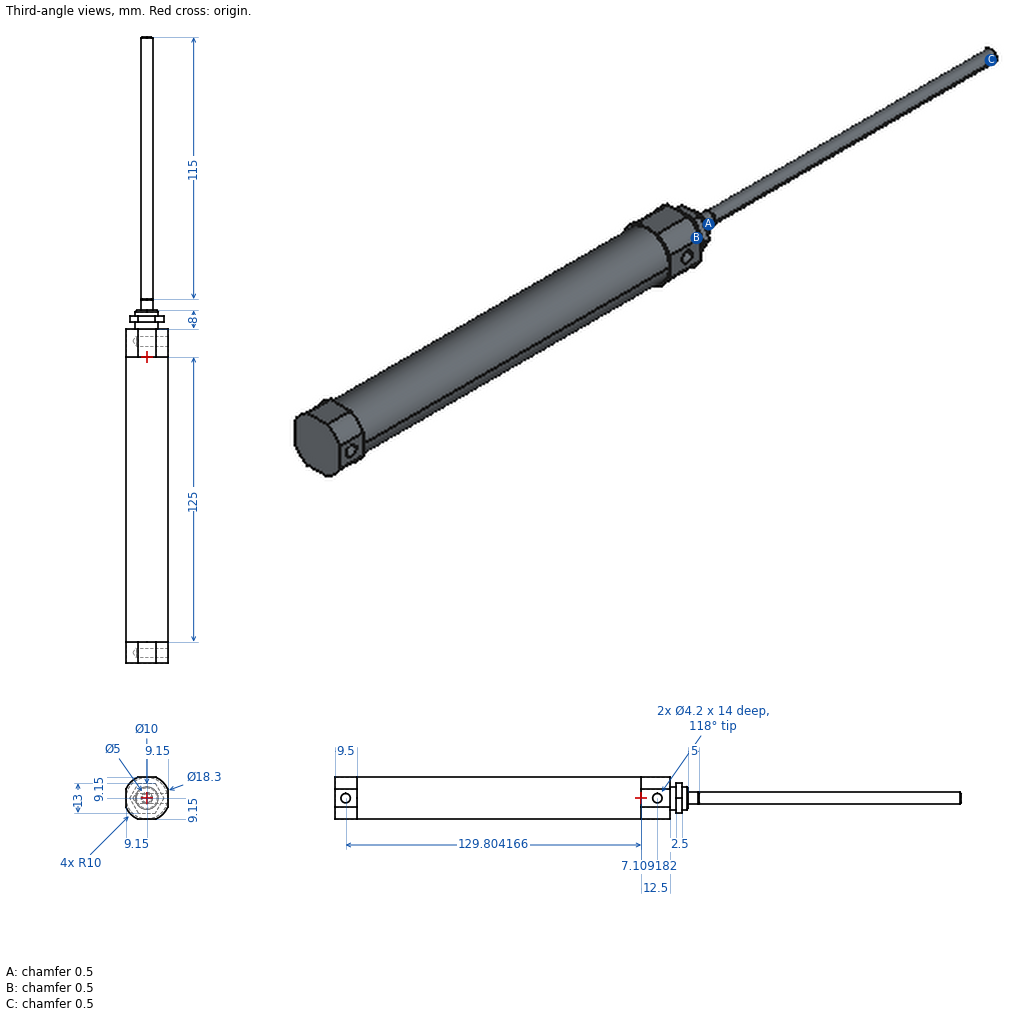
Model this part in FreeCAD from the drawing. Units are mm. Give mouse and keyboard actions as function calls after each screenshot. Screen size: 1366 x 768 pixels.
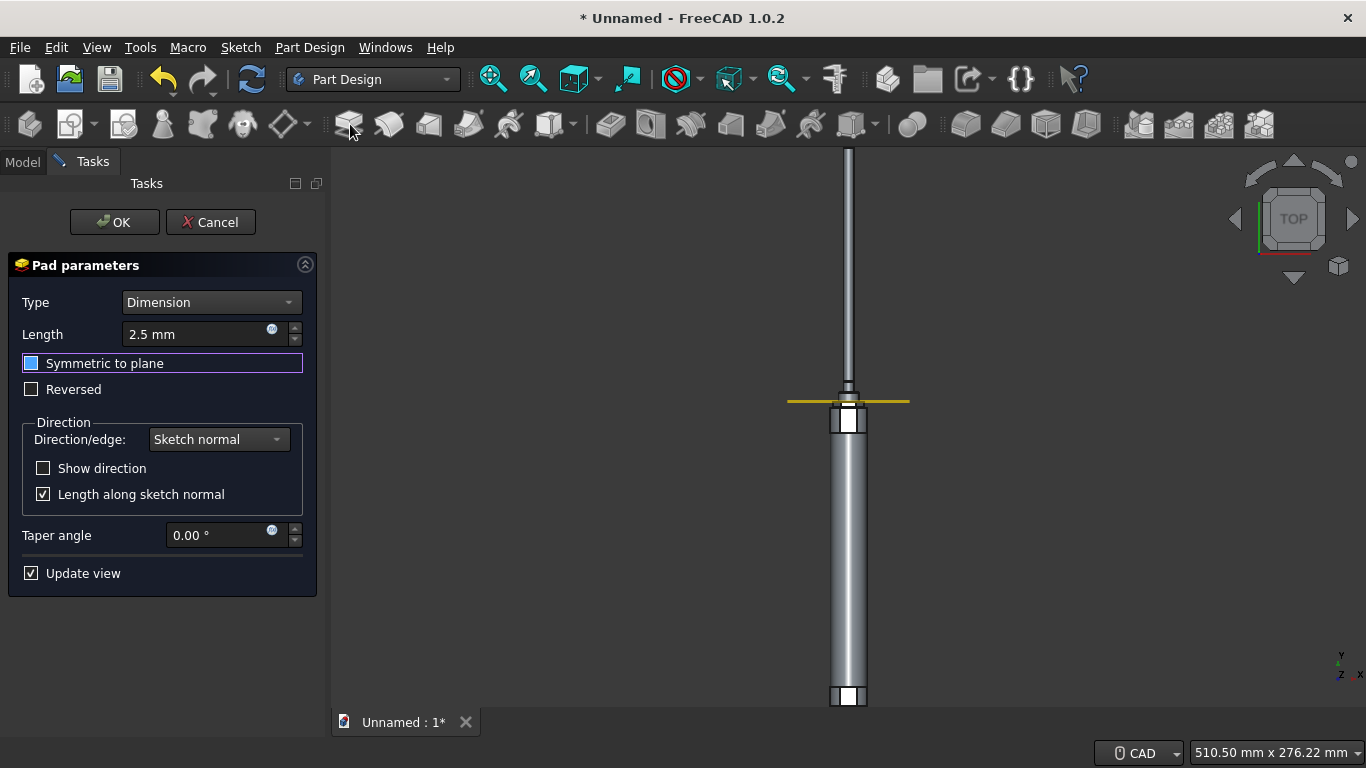
click(30, 389)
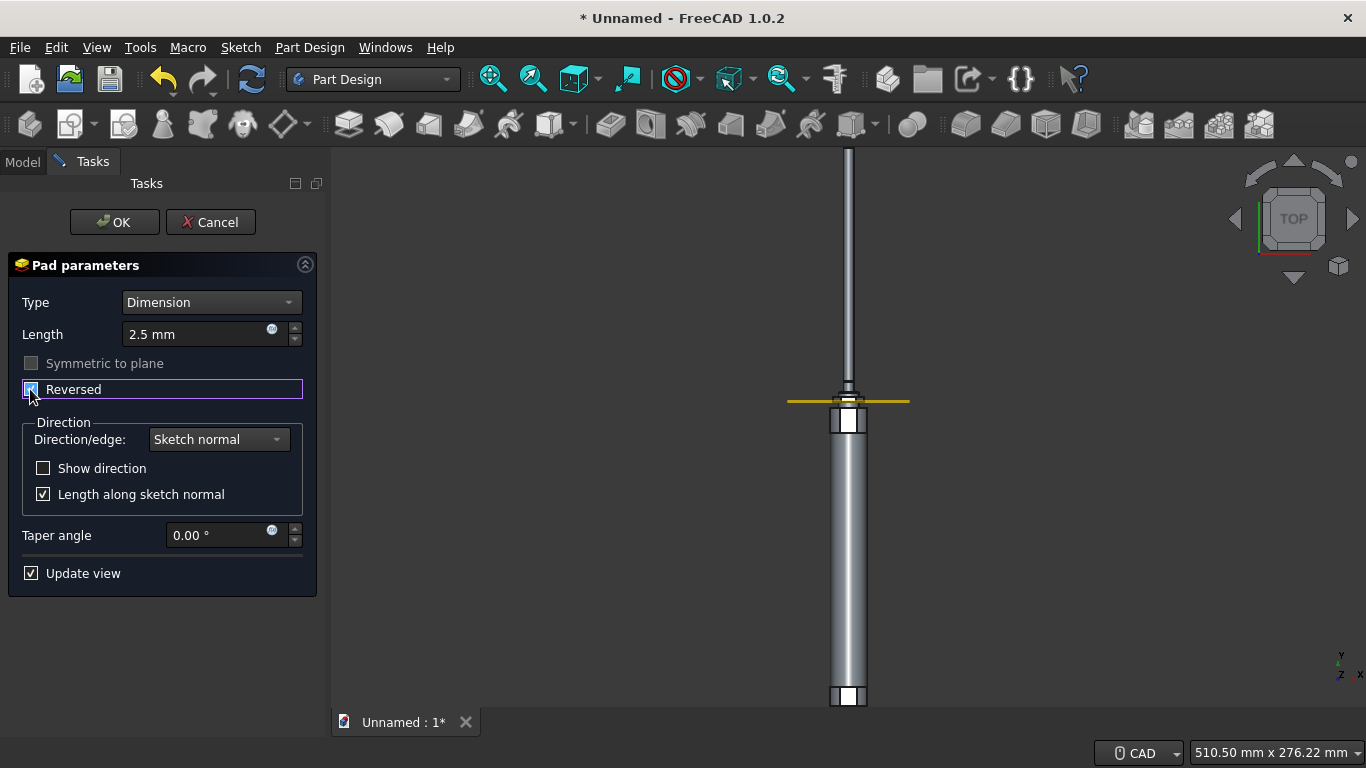
click(115, 222)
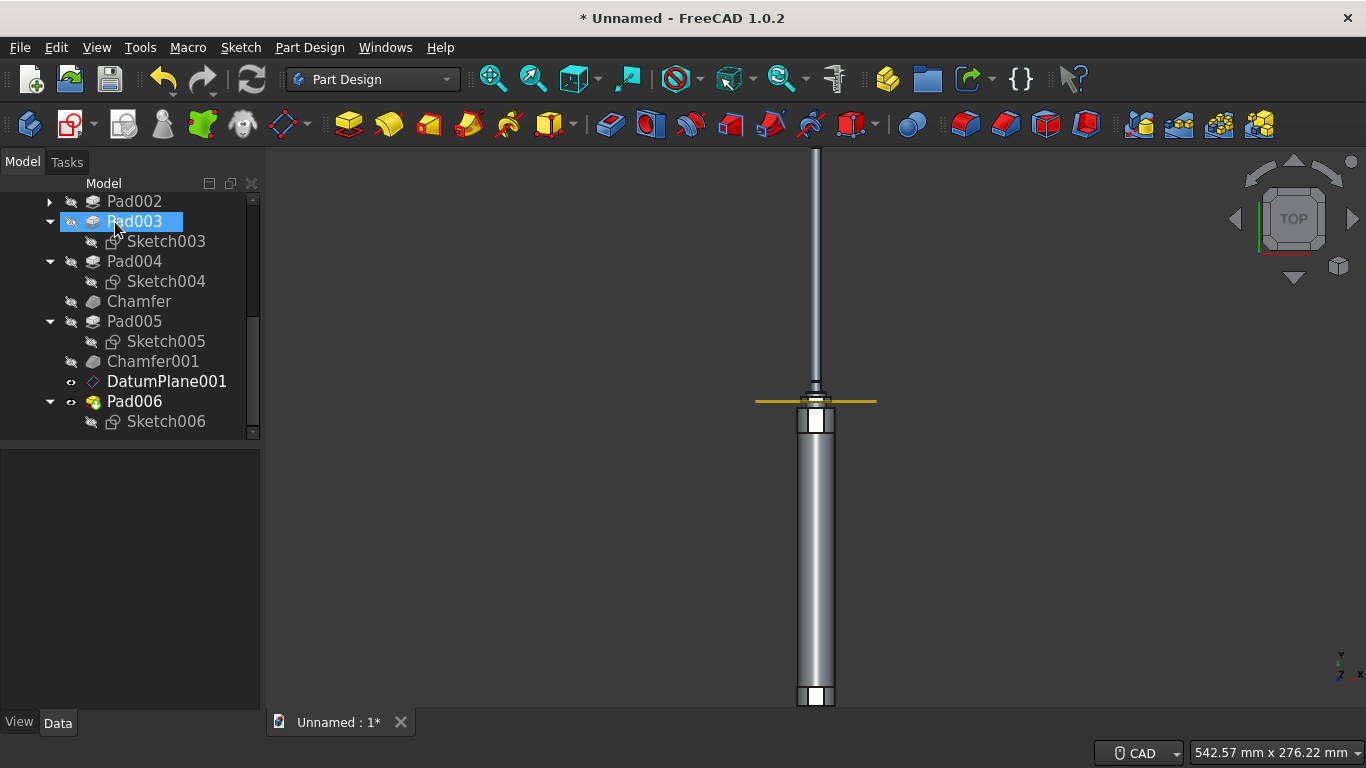
click(116, 382)
key(space)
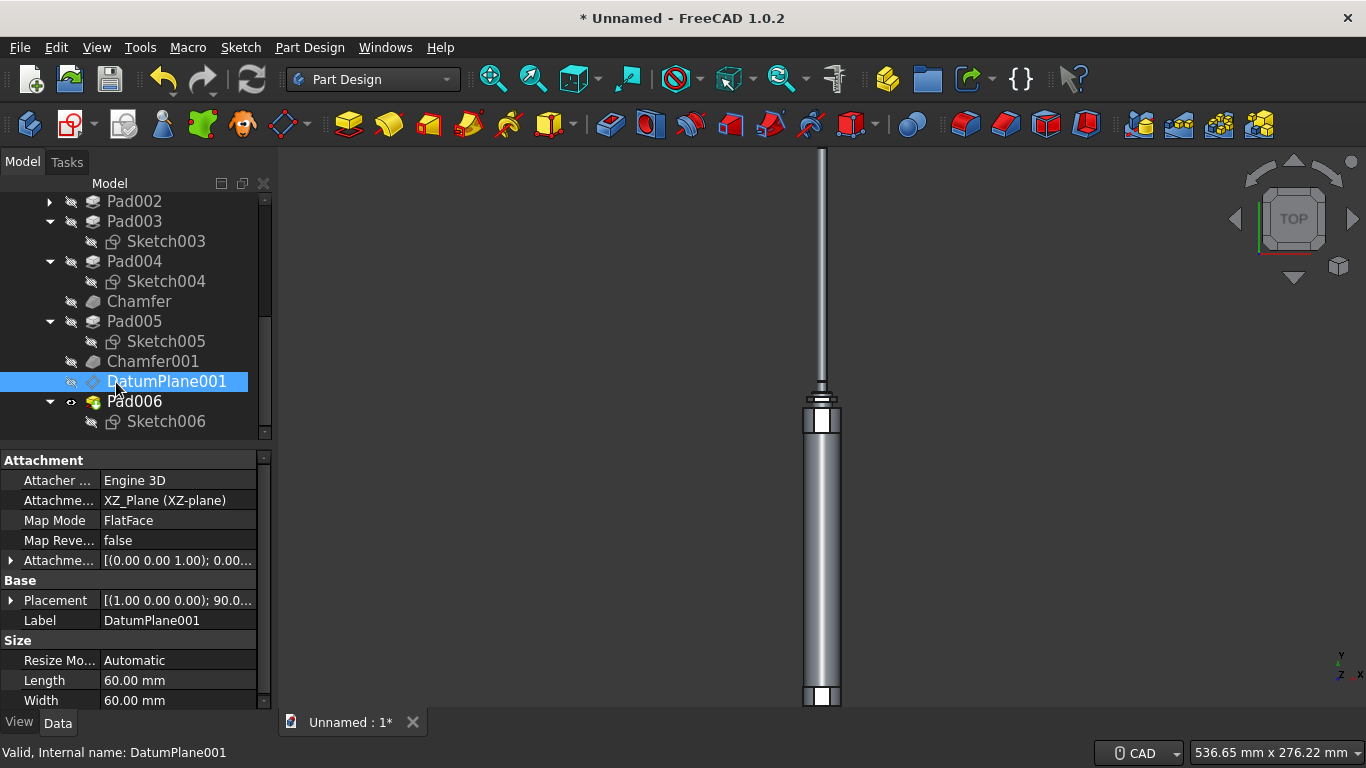
key(0)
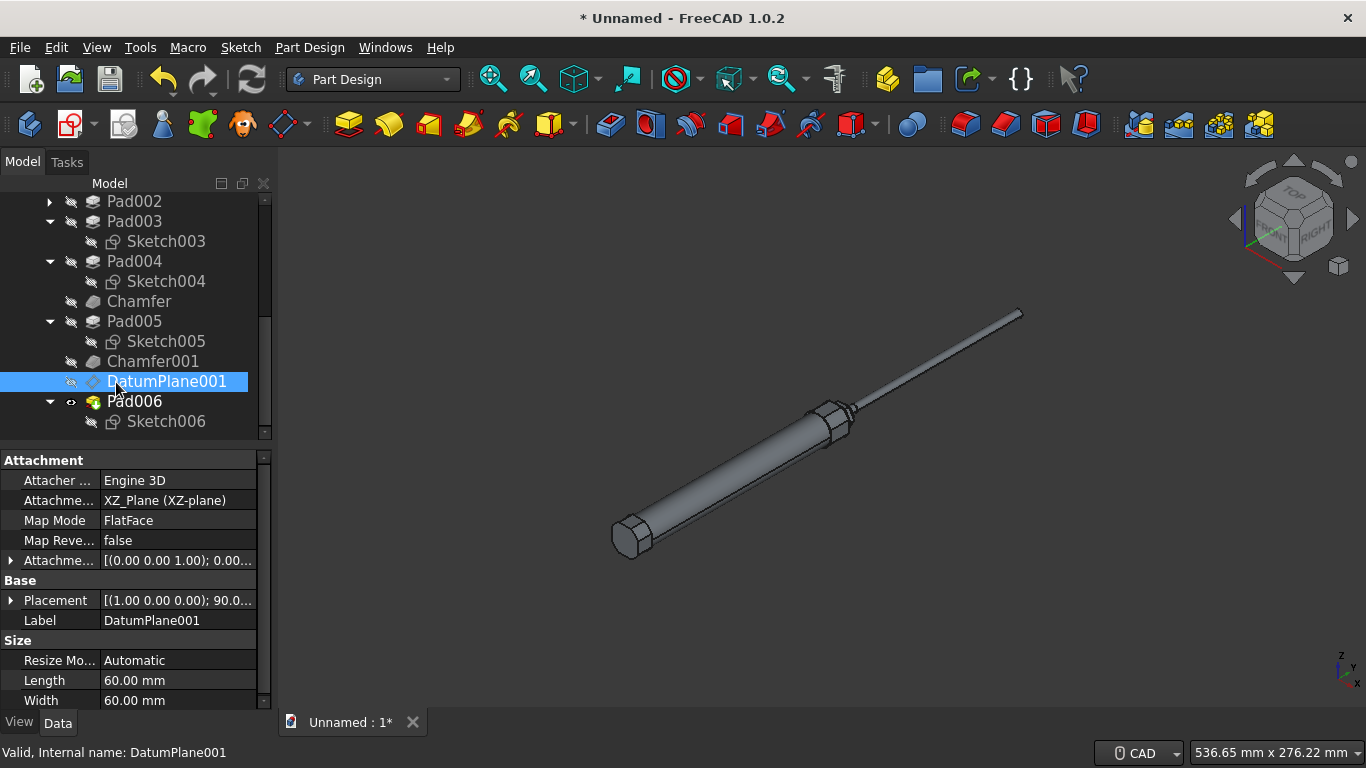
key(2)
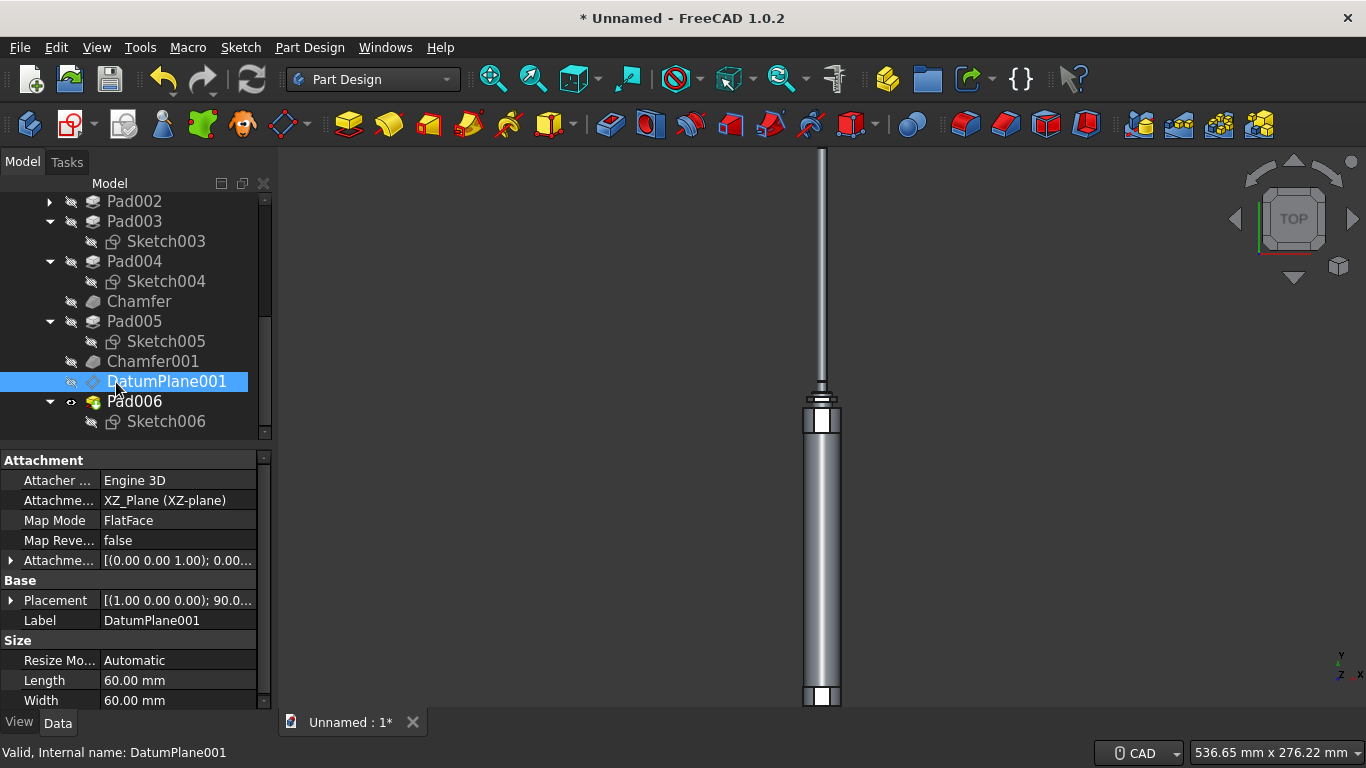
key(1)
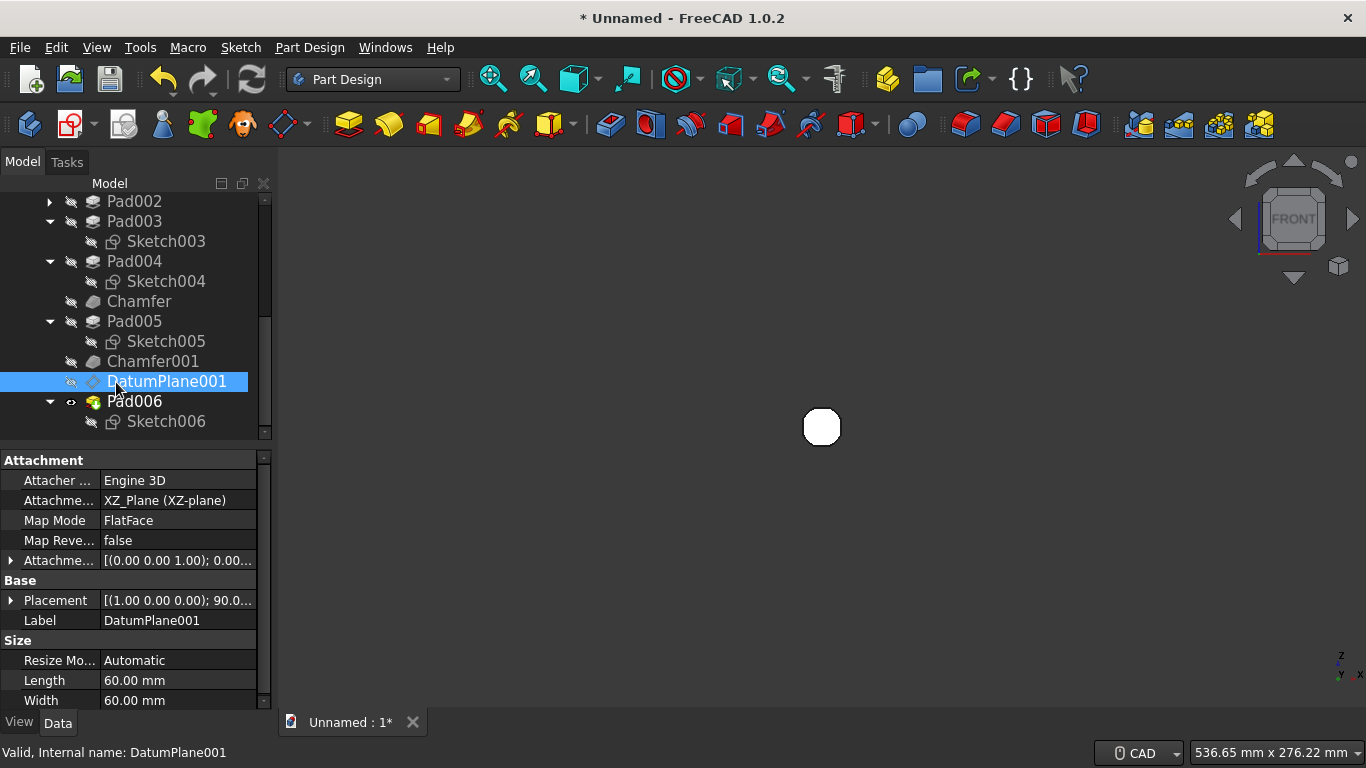
click(494, 80)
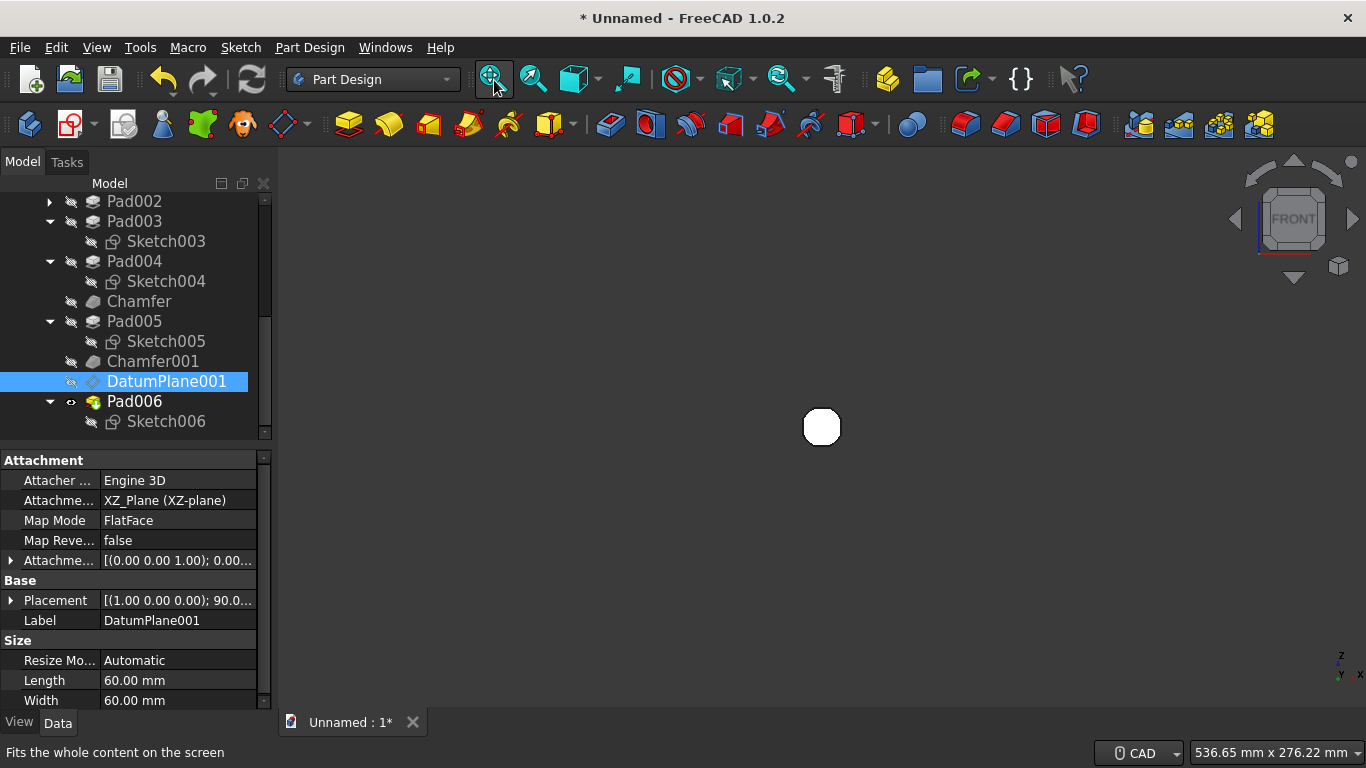
key(3)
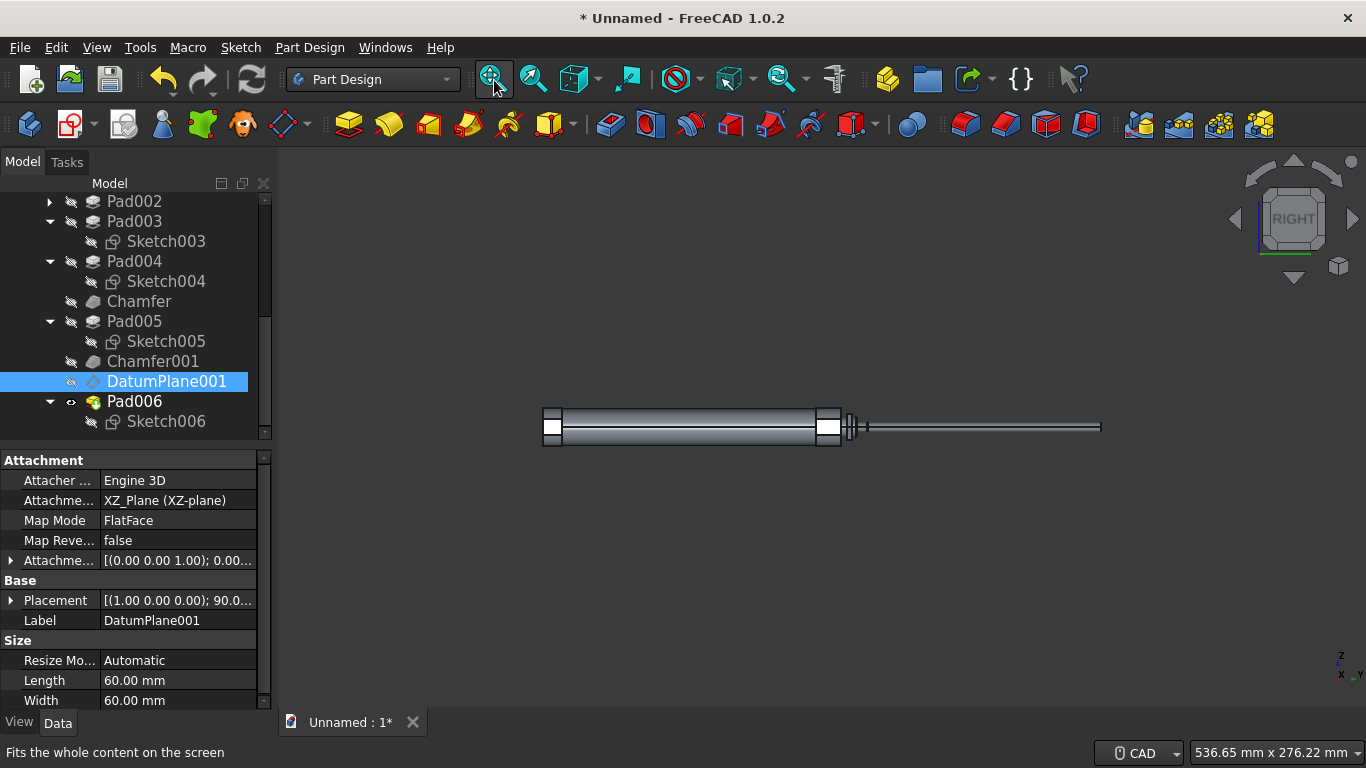
key(5)